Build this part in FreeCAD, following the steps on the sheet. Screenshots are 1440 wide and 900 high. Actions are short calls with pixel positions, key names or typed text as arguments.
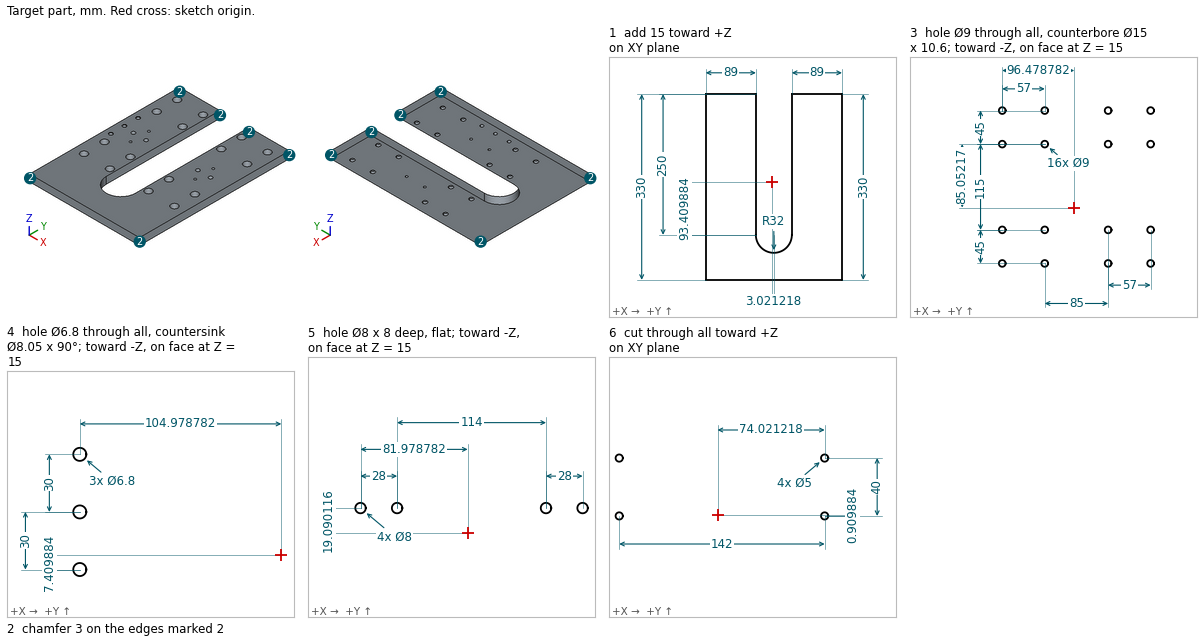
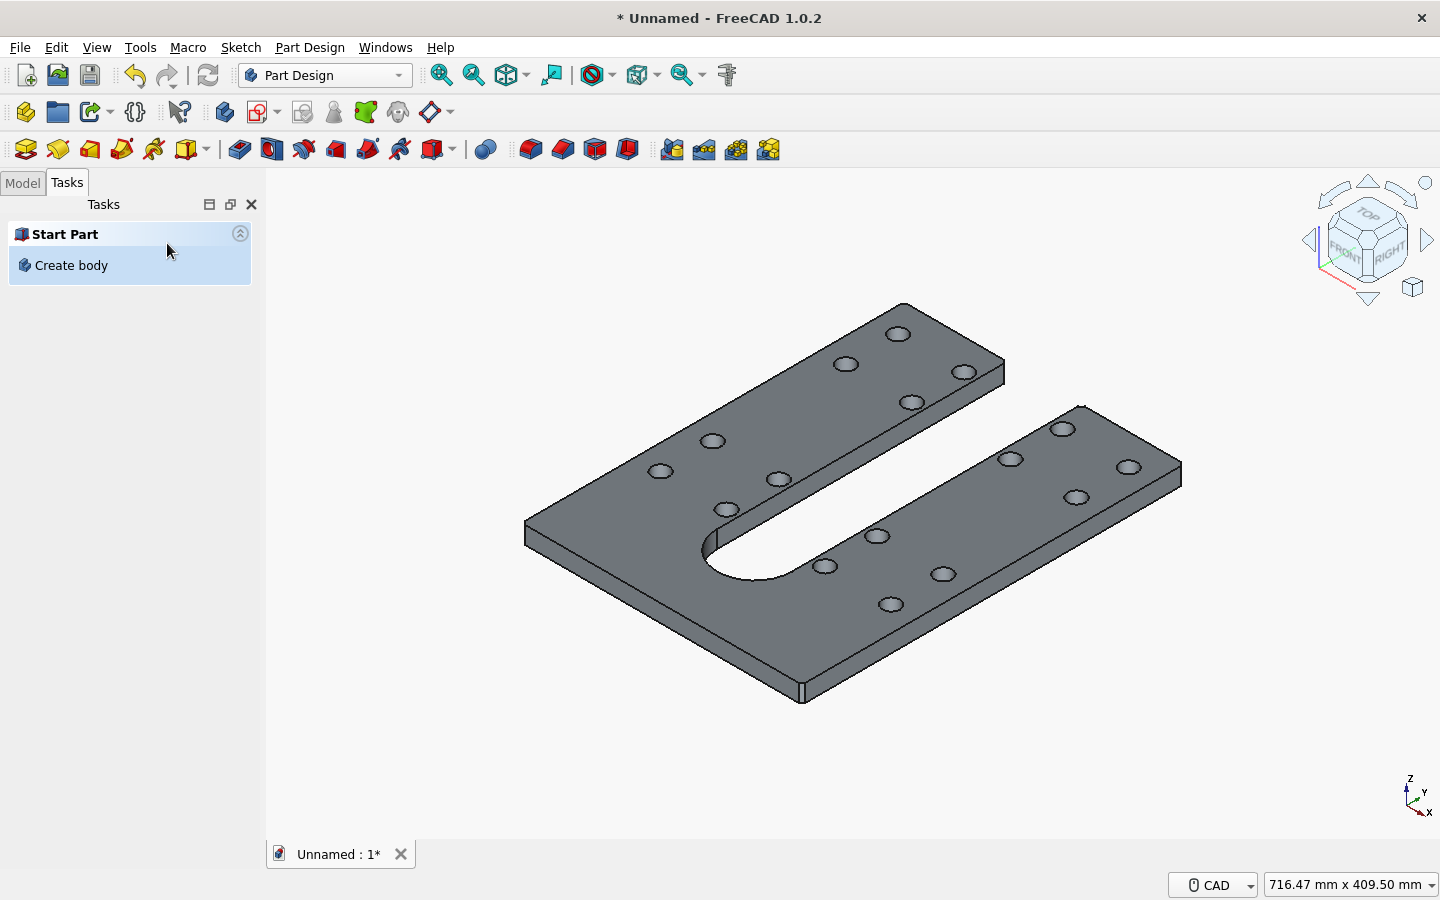
click(988, 507)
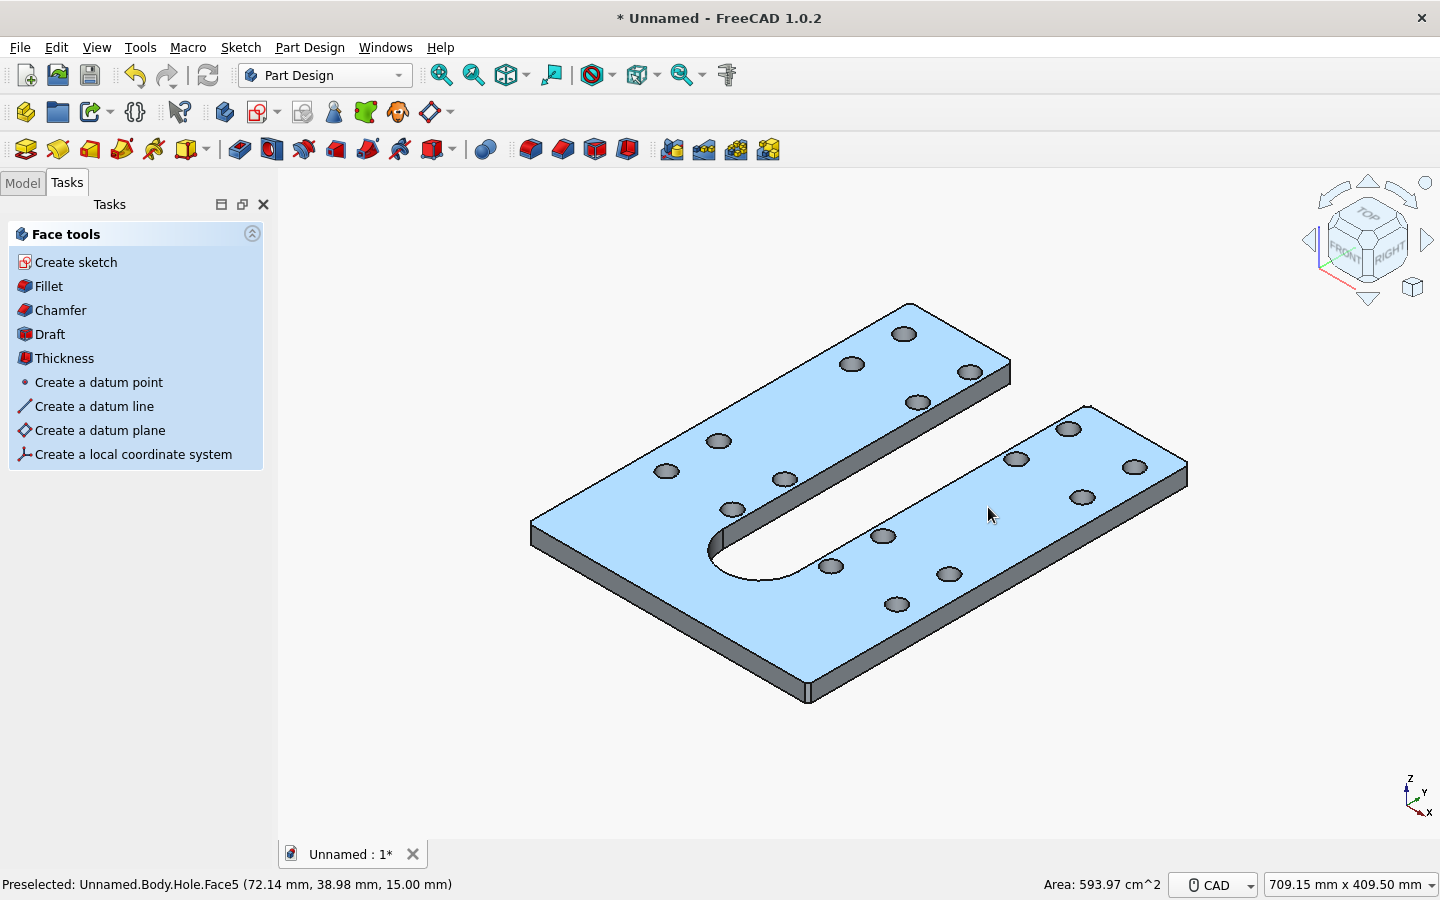
click(258, 112)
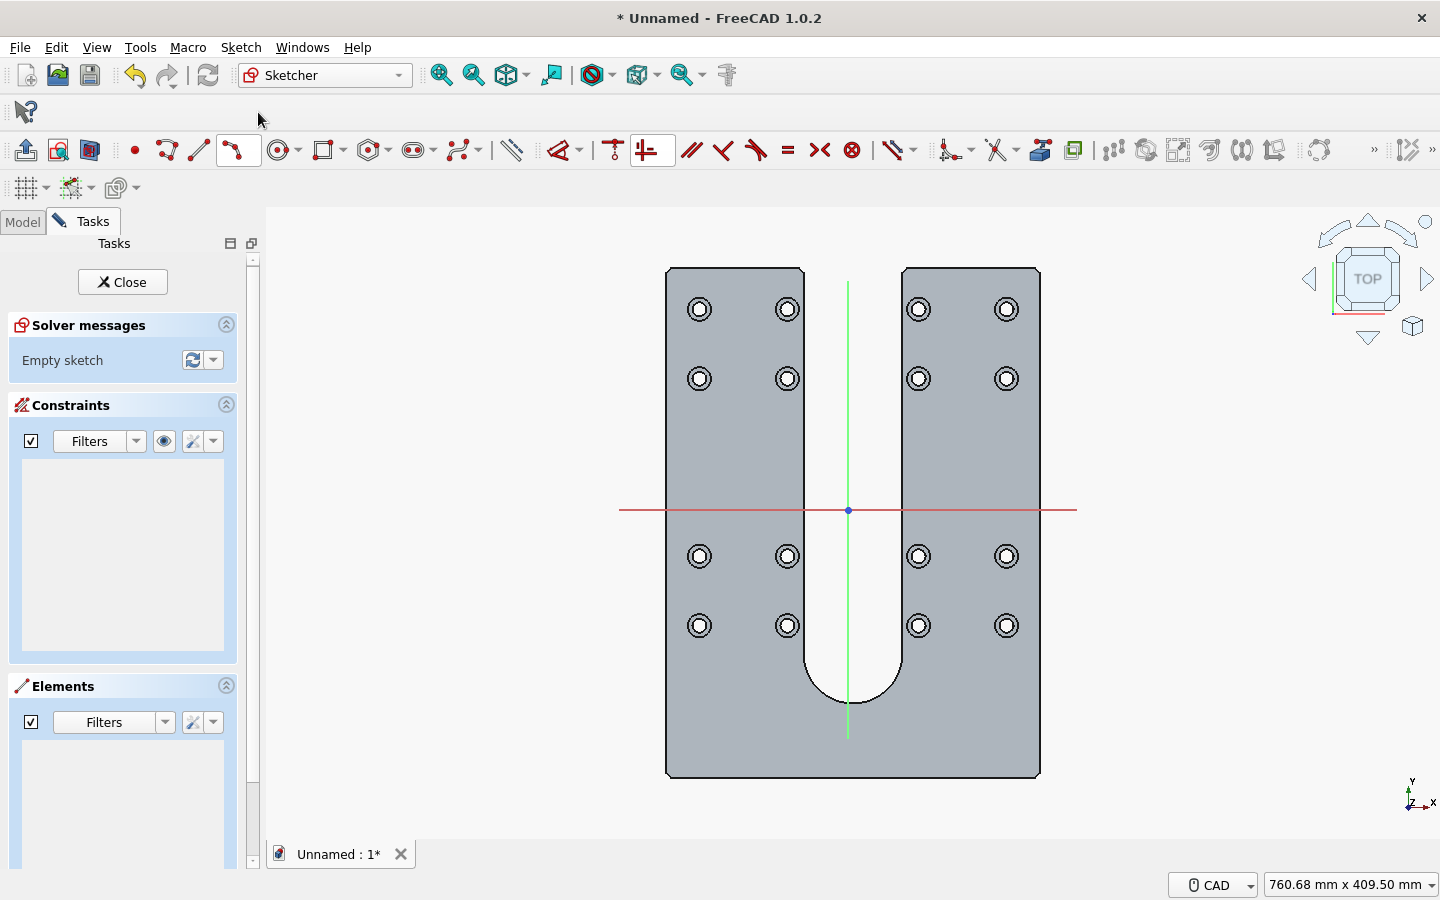
scroll(758, 459, up, 7)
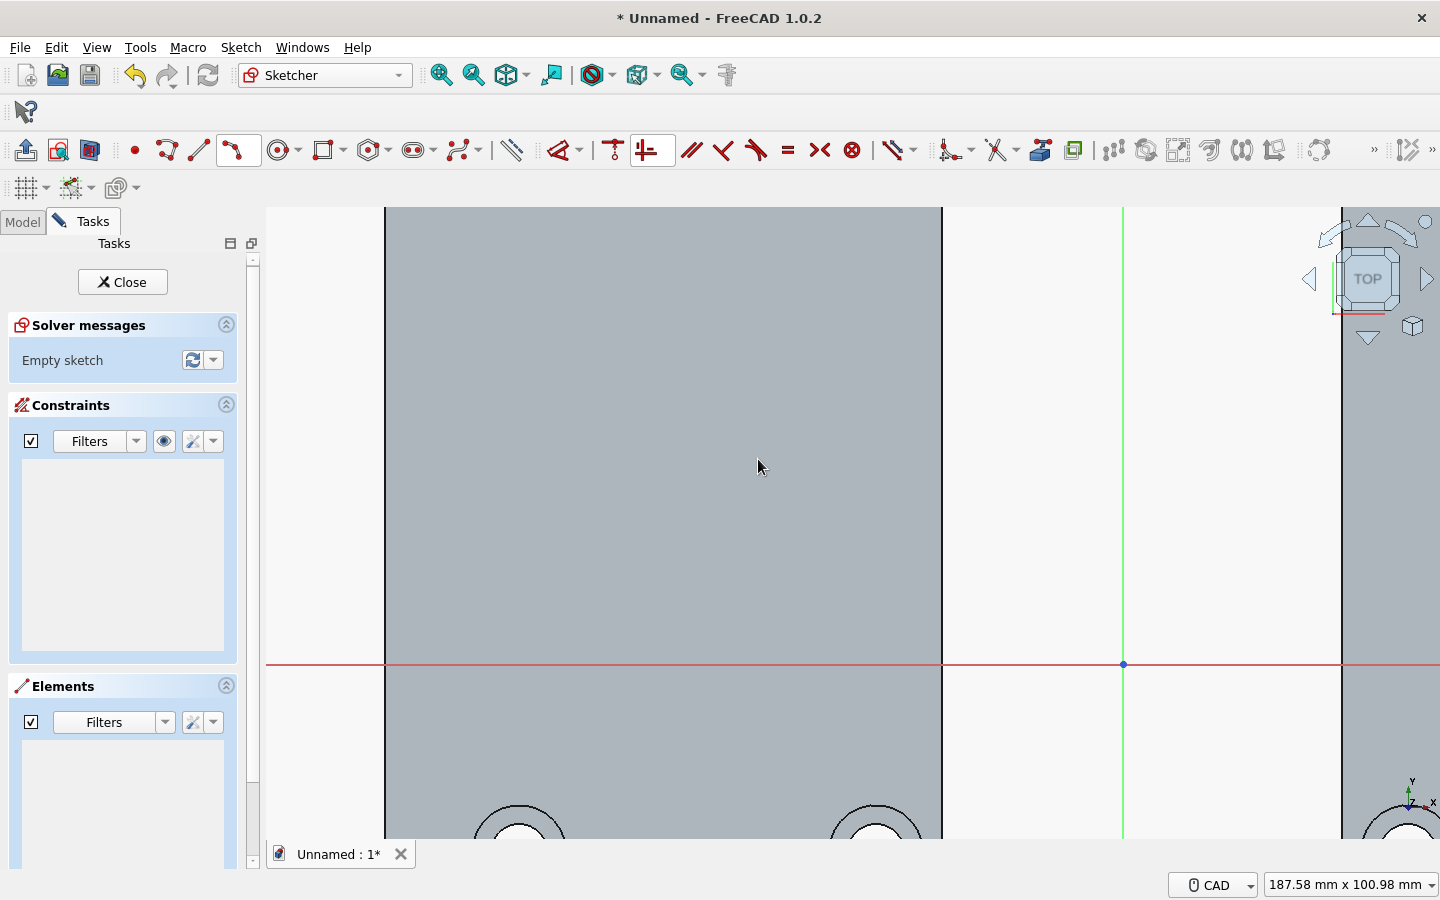
click(278, 150)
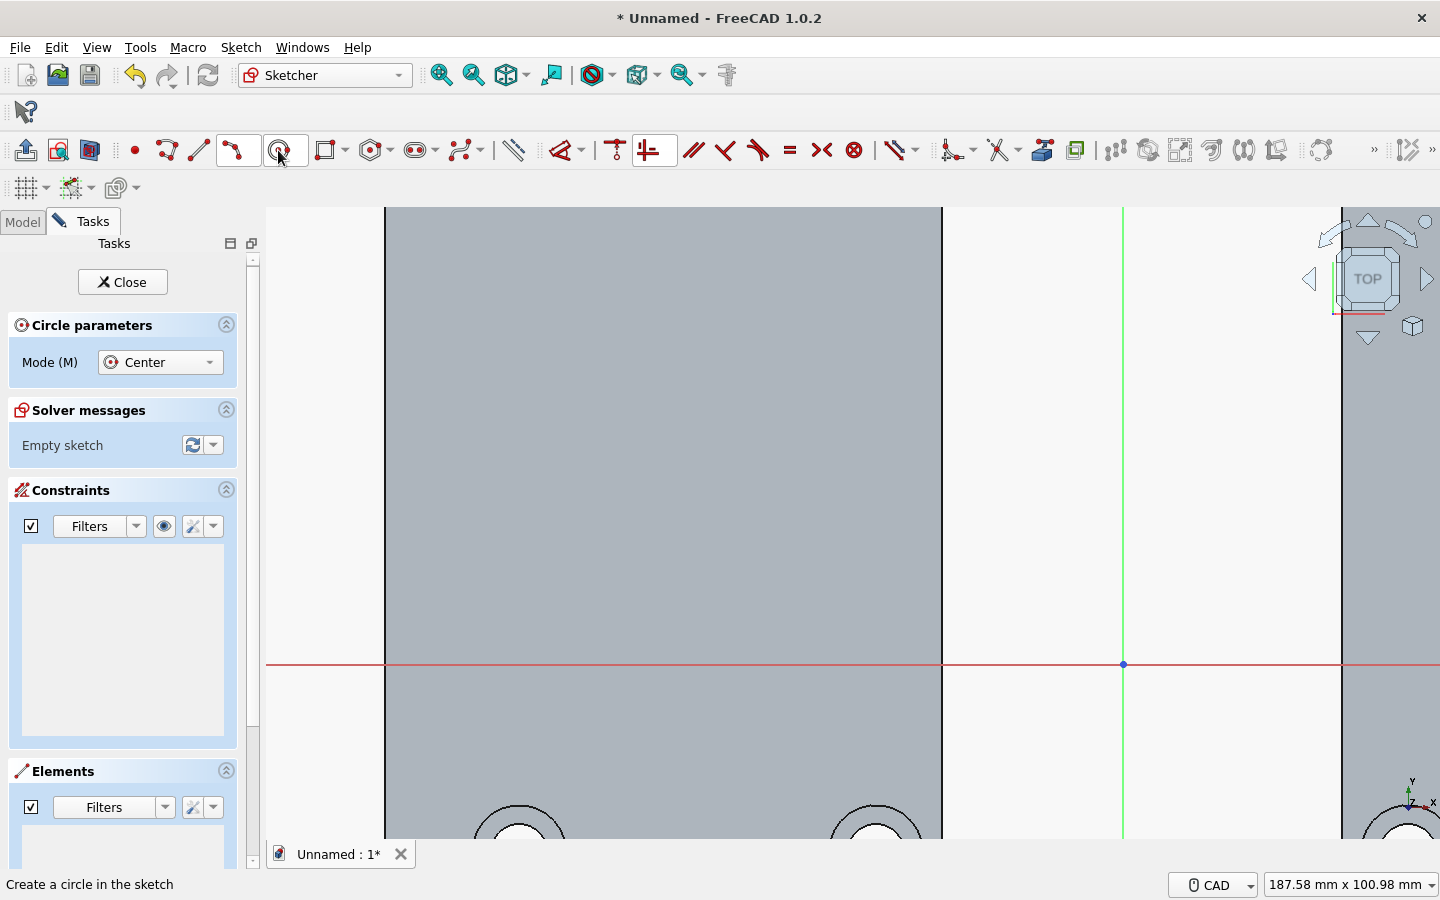
click(466, 336)
move(481, 320)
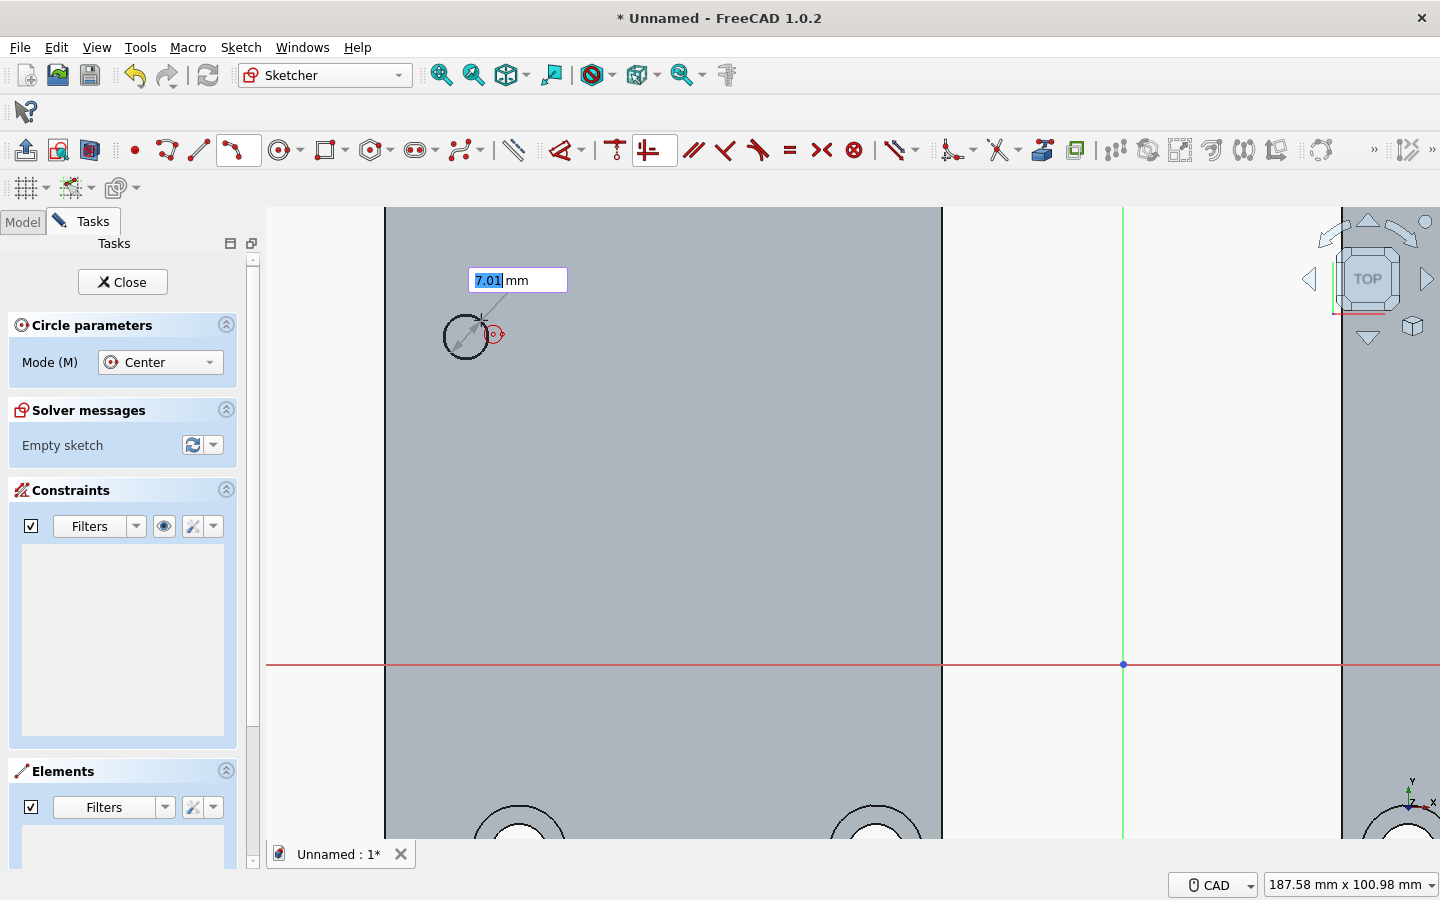
text(6.8)
key(Return)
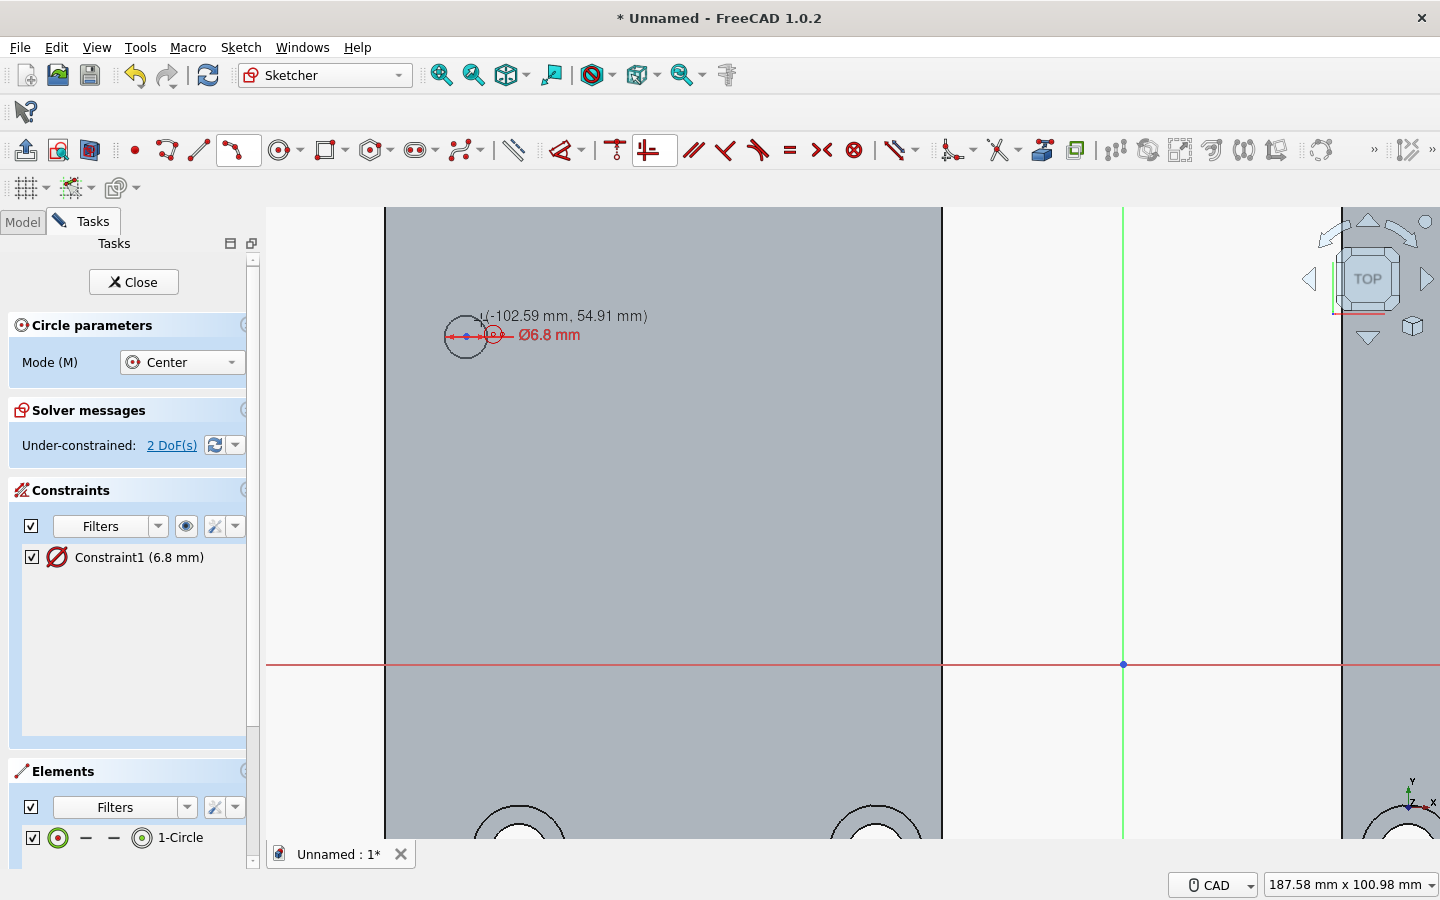
click(466, 523)
move(481, 508)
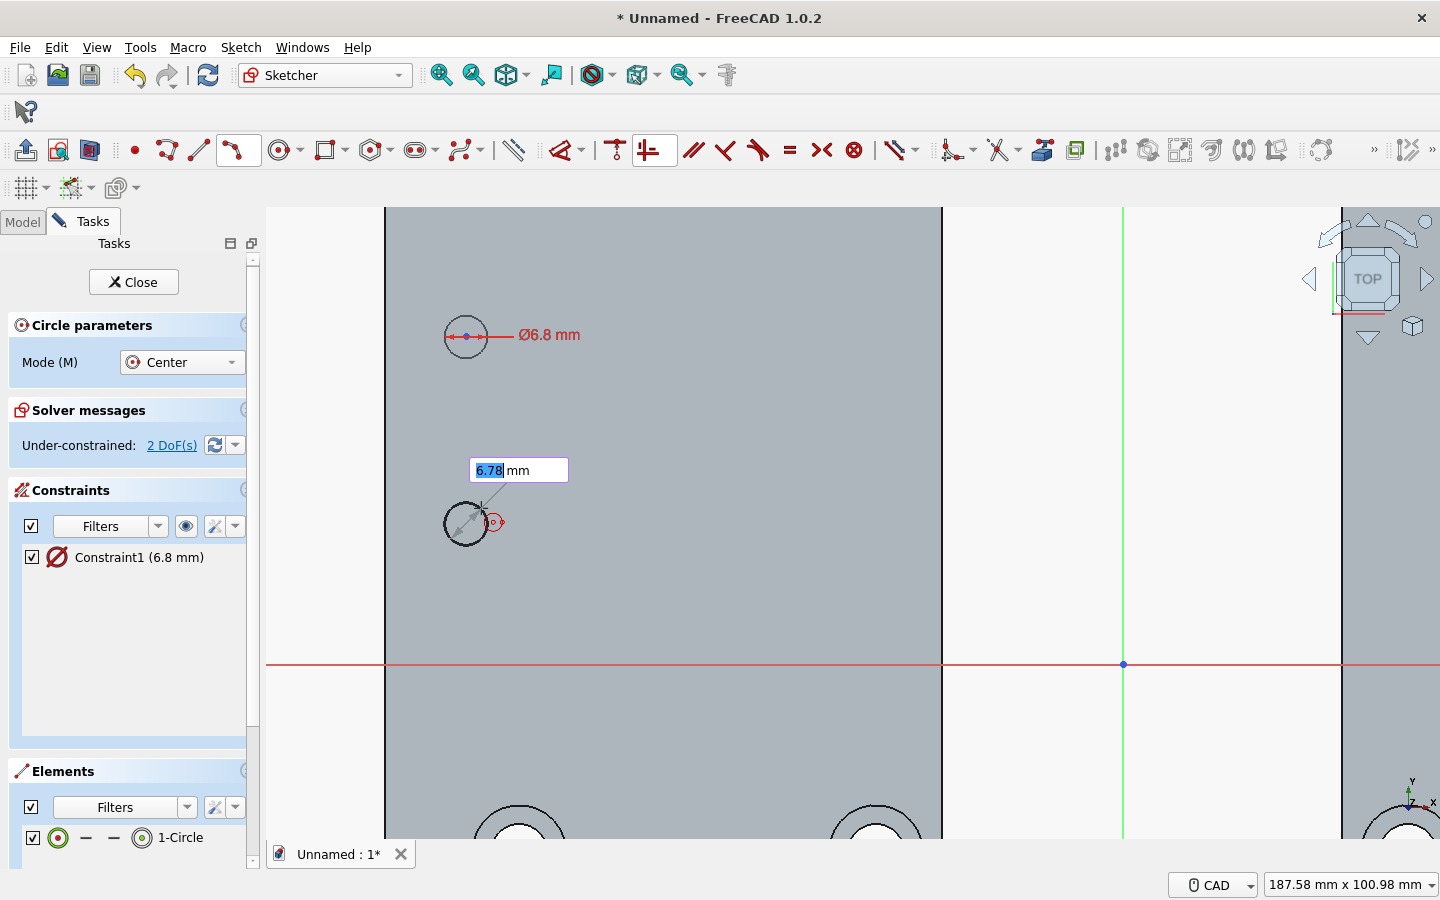
text(6.8)
key(Return)